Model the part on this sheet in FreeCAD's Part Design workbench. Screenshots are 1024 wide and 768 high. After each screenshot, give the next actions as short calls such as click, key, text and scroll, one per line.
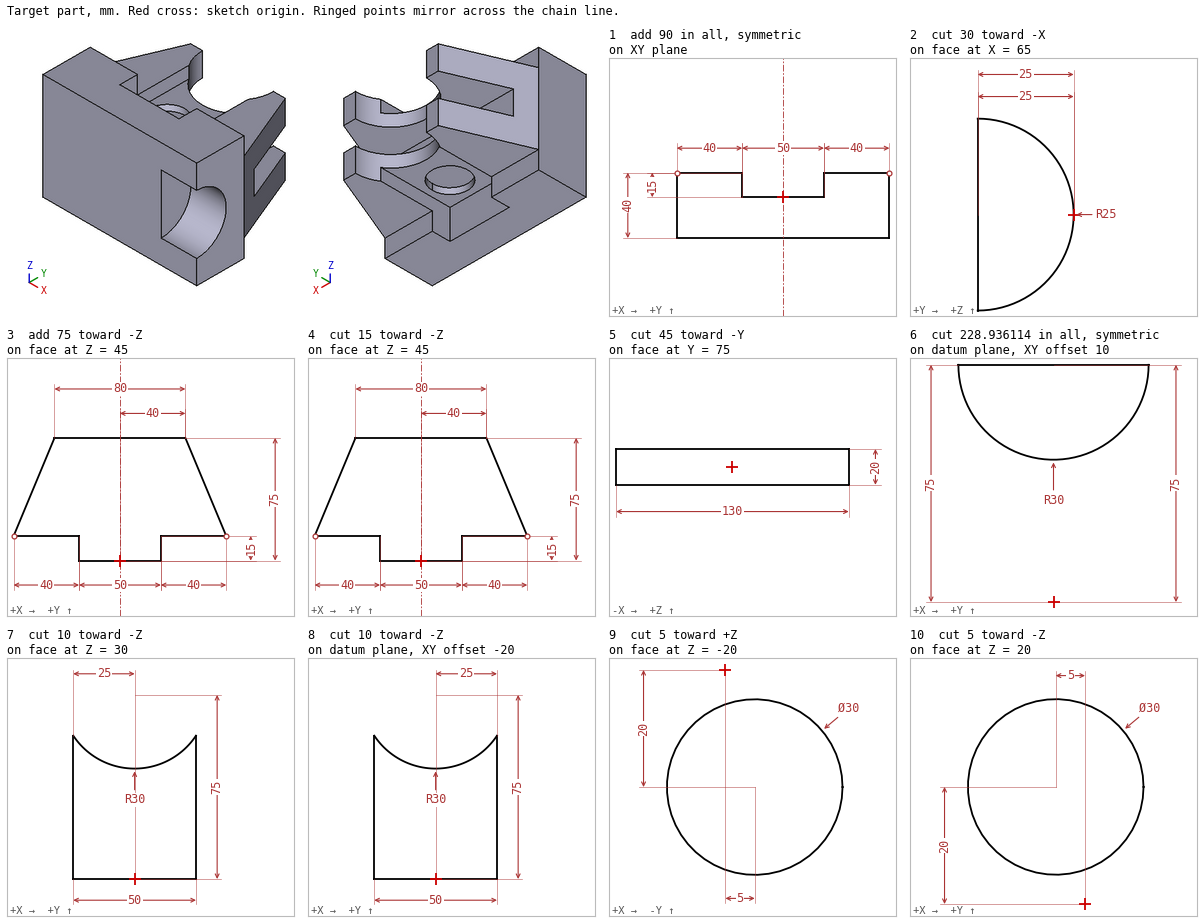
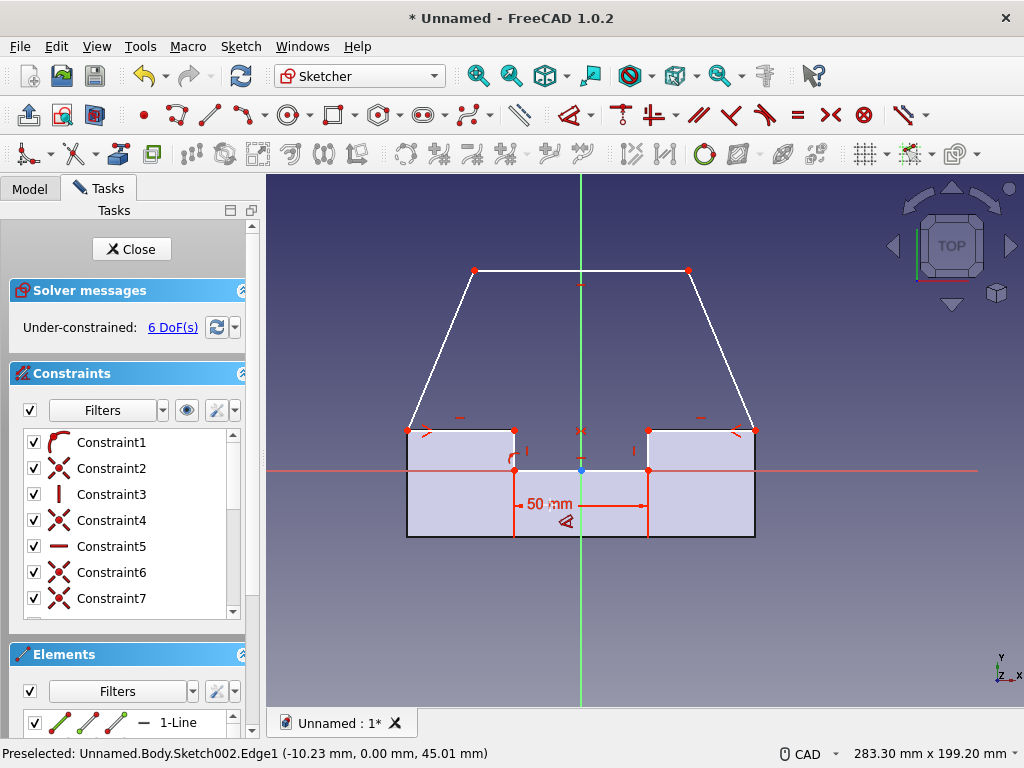
click(648, 459)
click(682, 451)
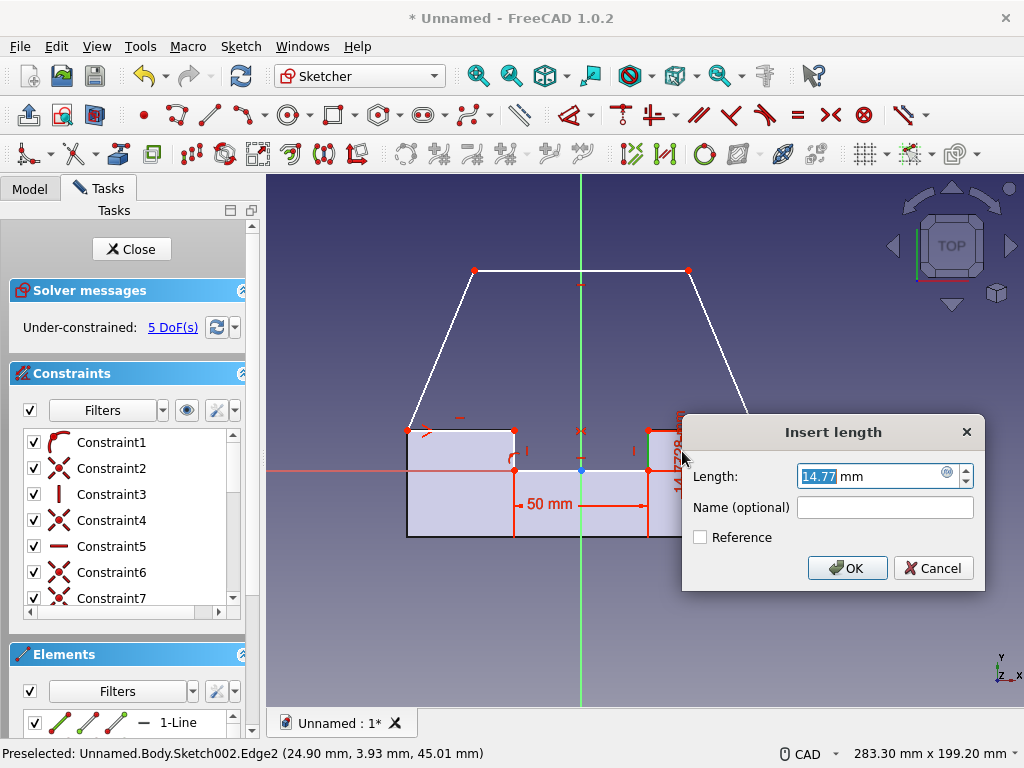
text(15)
key(Return)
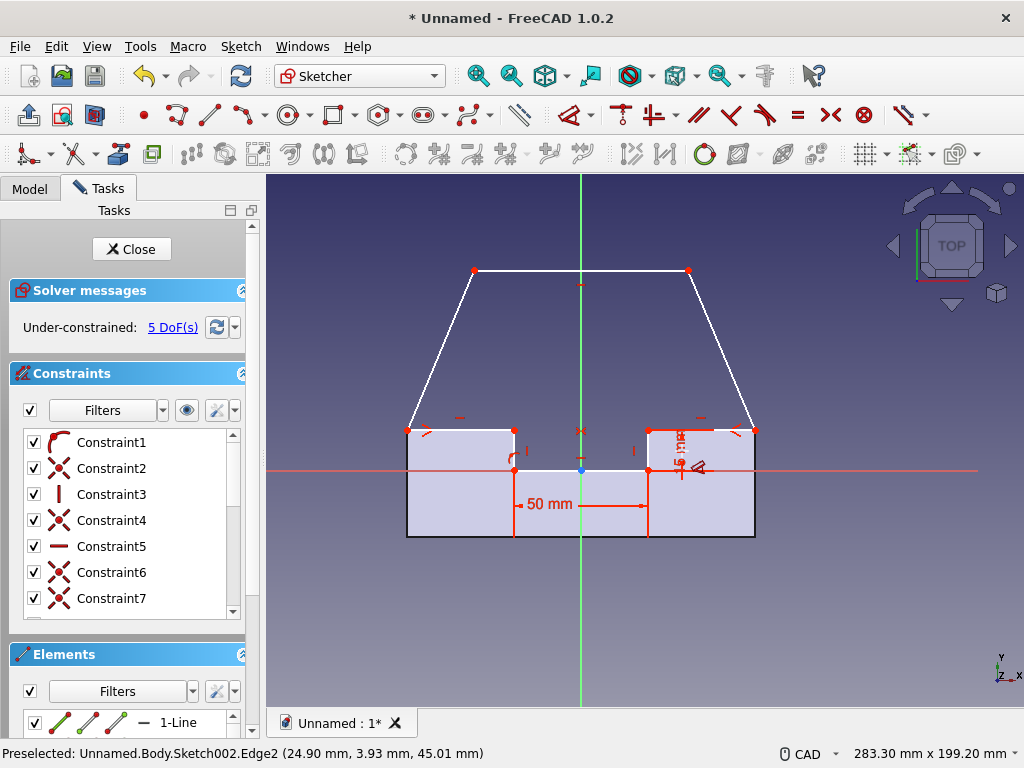
click(680, 430)
click(702, 396)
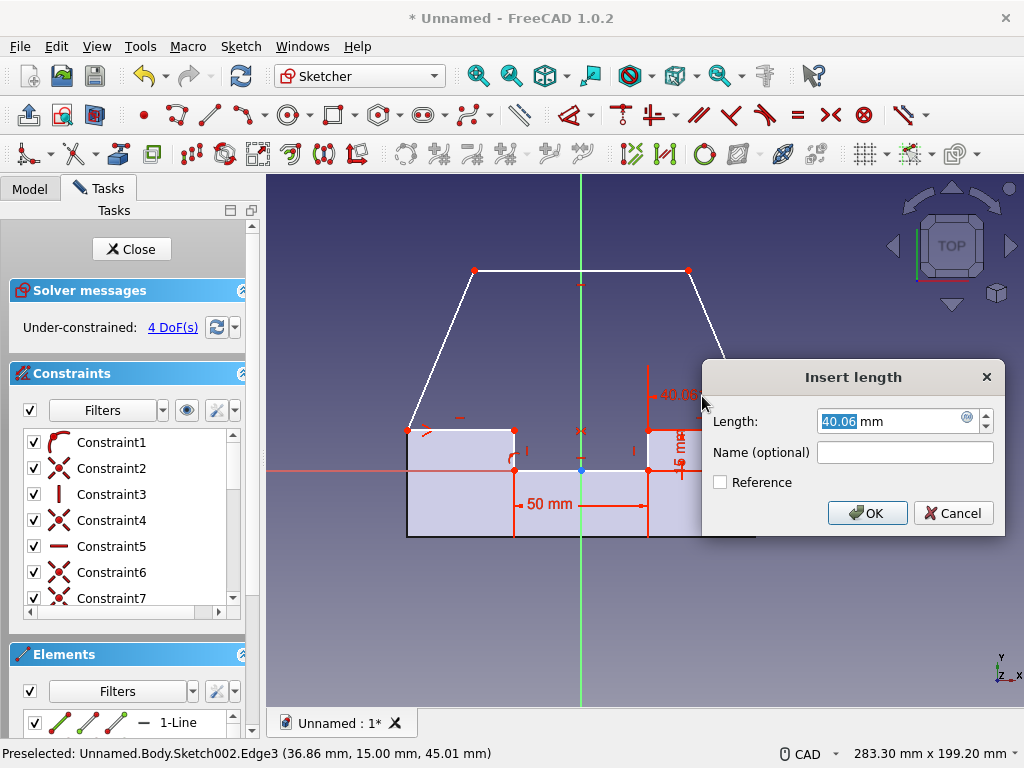
text(40)
key(Return)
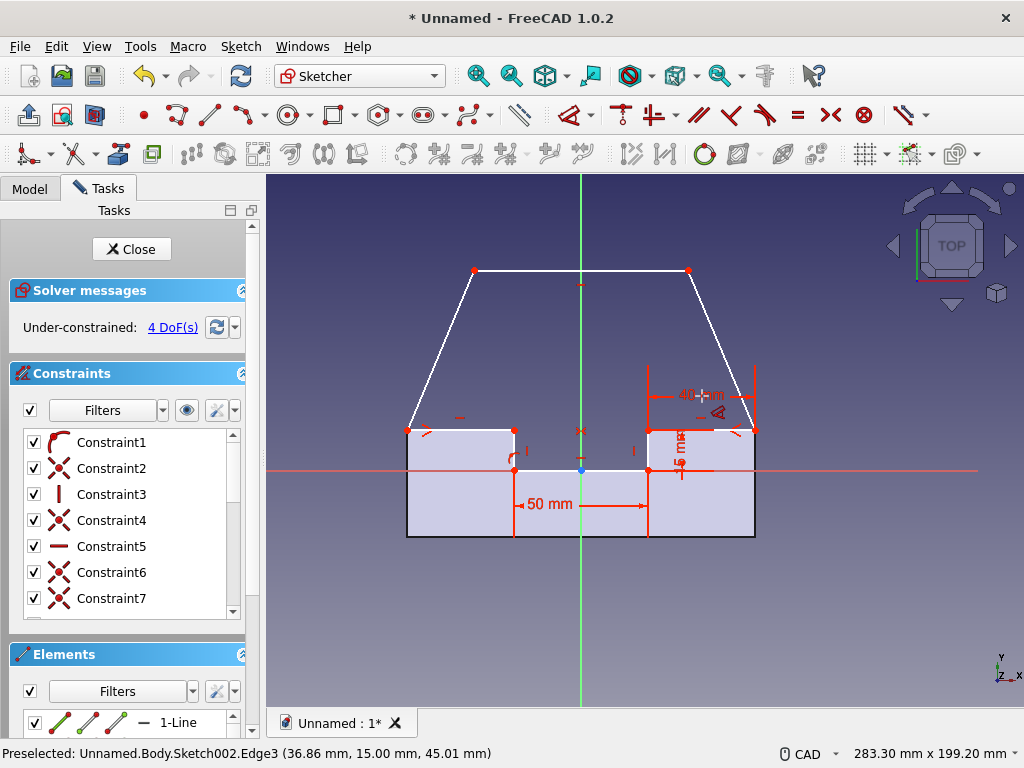
click(624, 271)
click(532, 237)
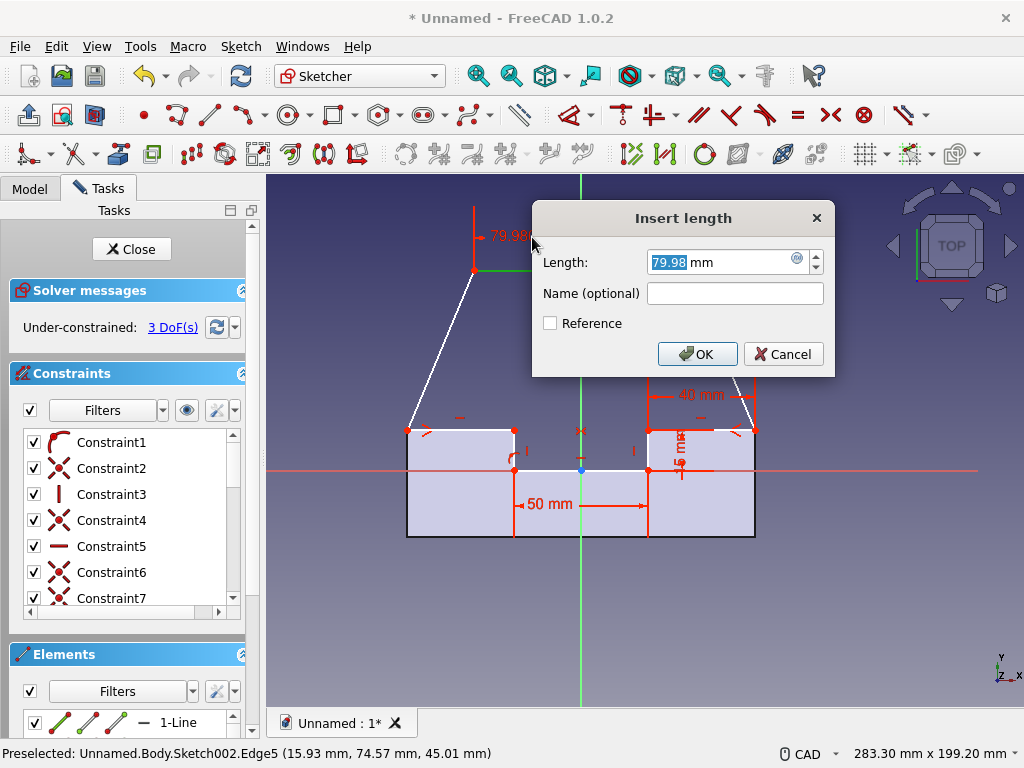
text(80)
key(Return)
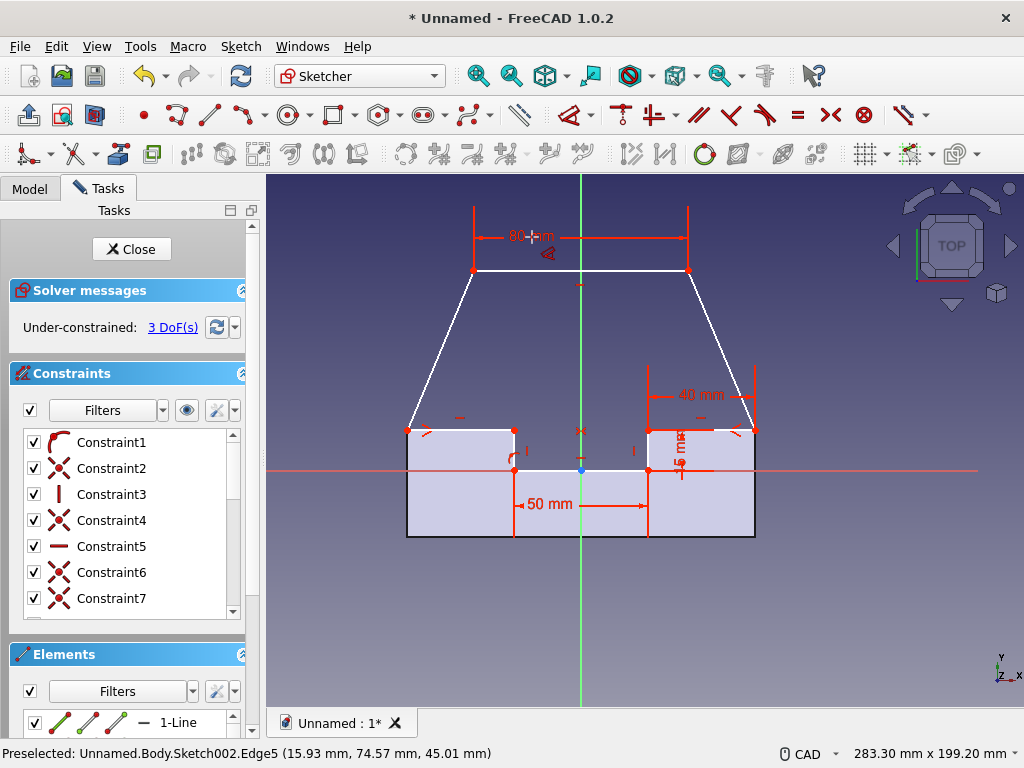
click(440, 430)
click(461, 396)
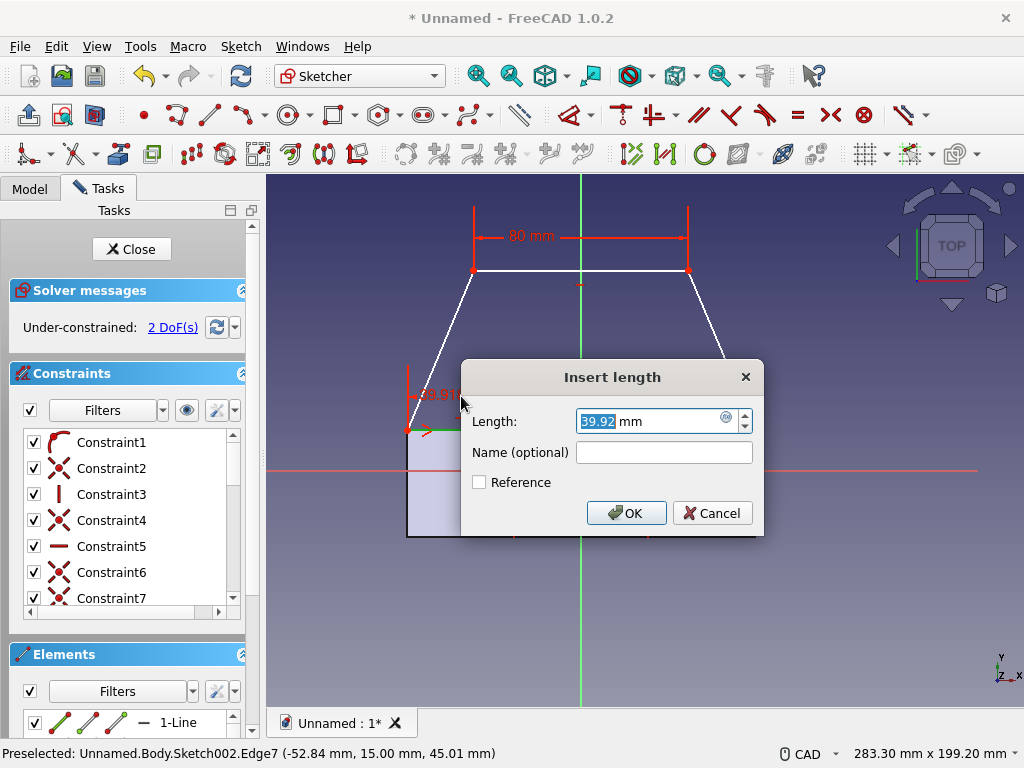
text(40)
key(Return)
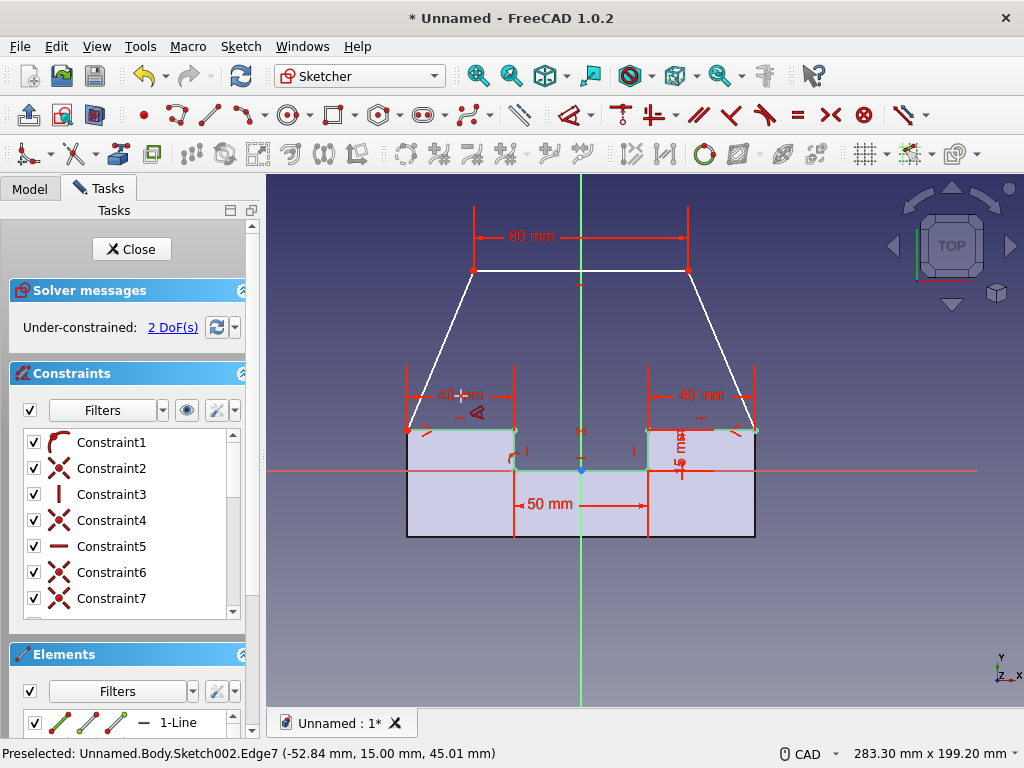
click(688, 271)
click(635, 505)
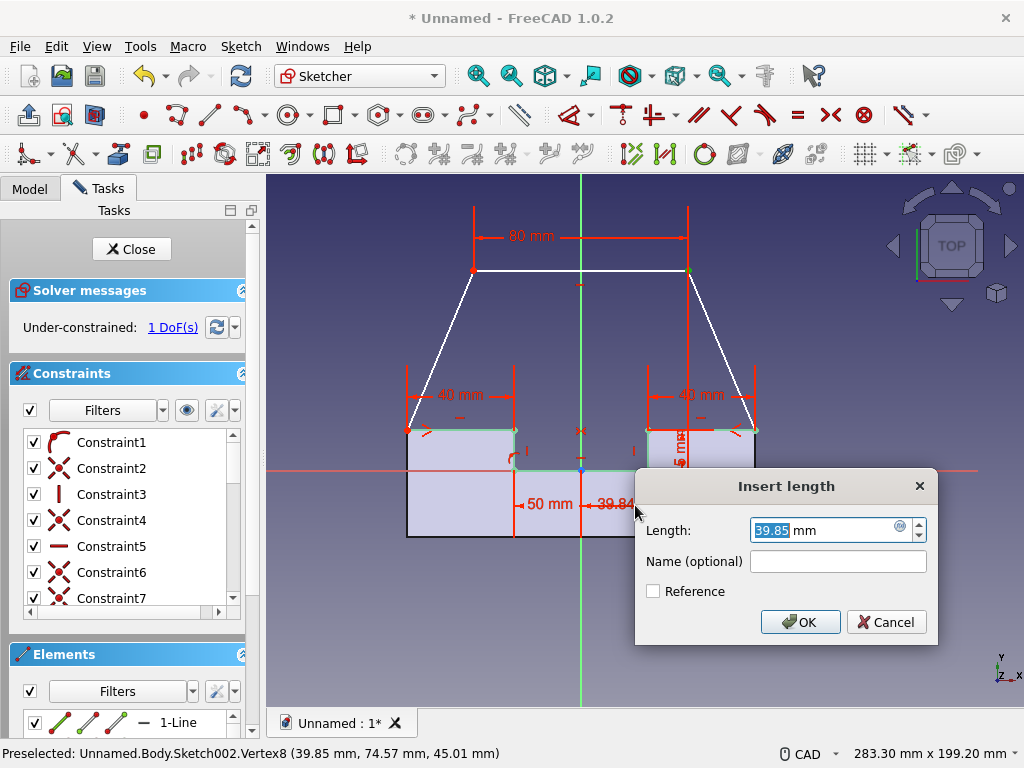
text(40)
key(Return)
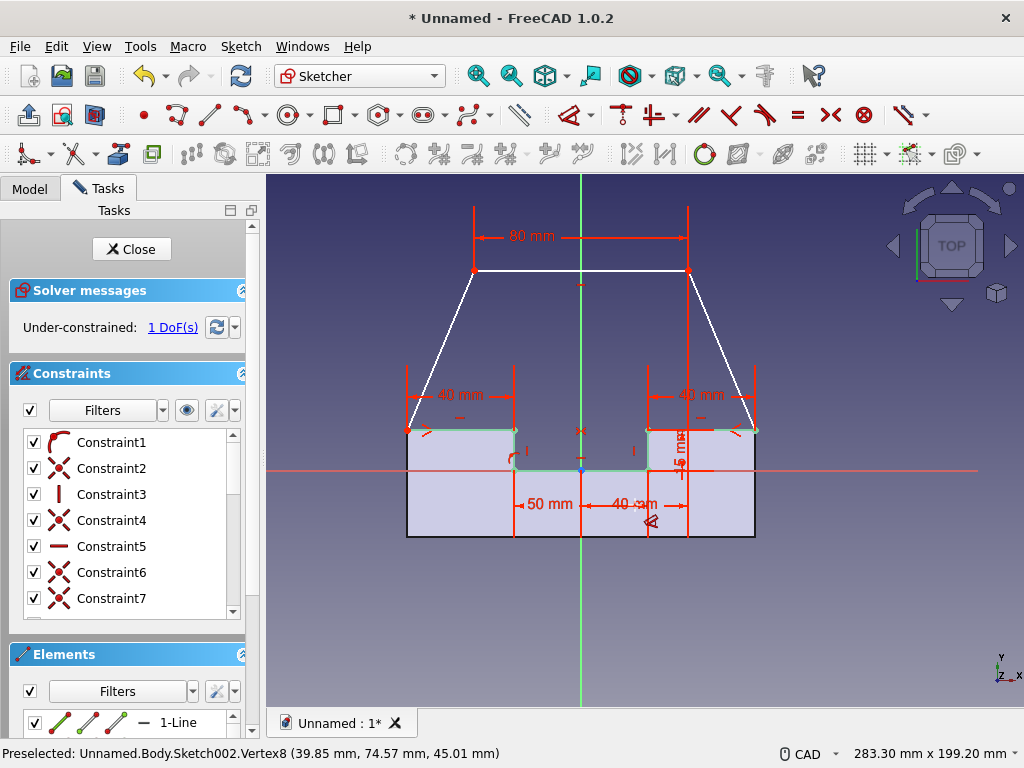
click(688, 271)
click(722, 417)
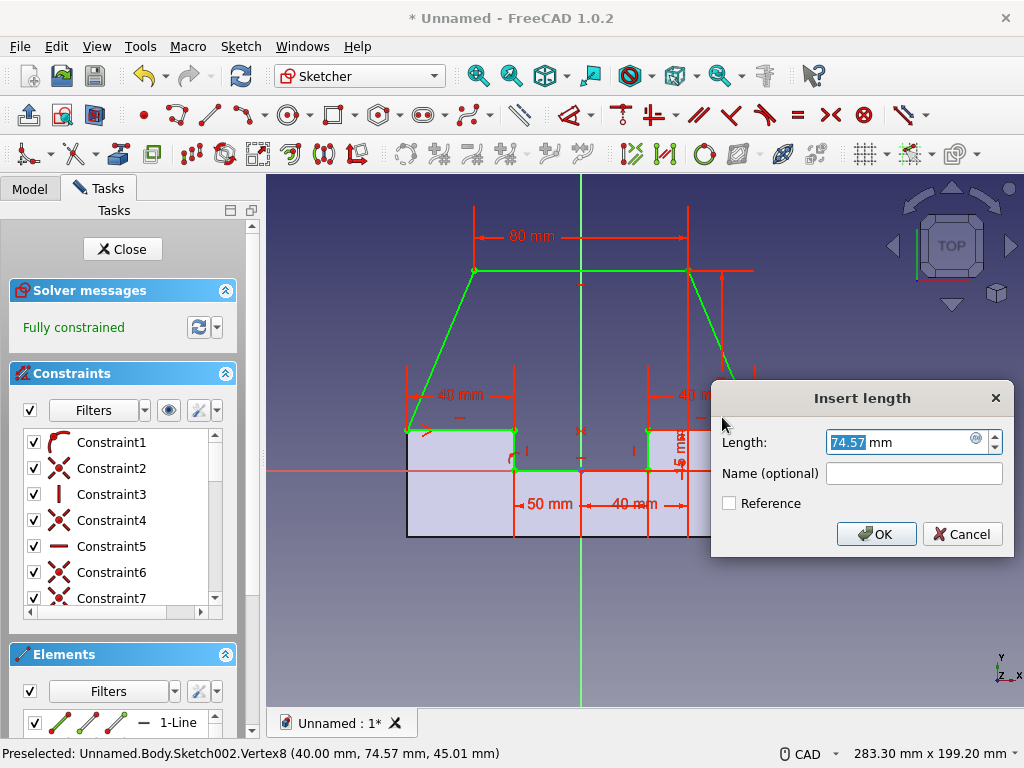
text(75)
key(Return)
key(Escape)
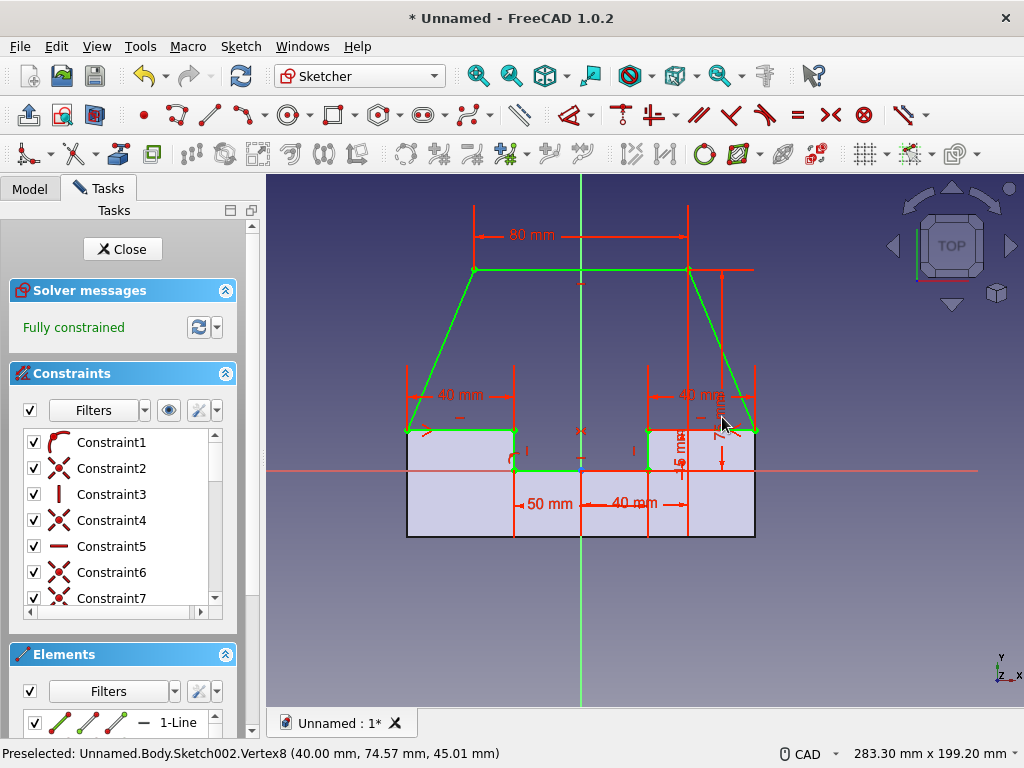
click(123, 249)